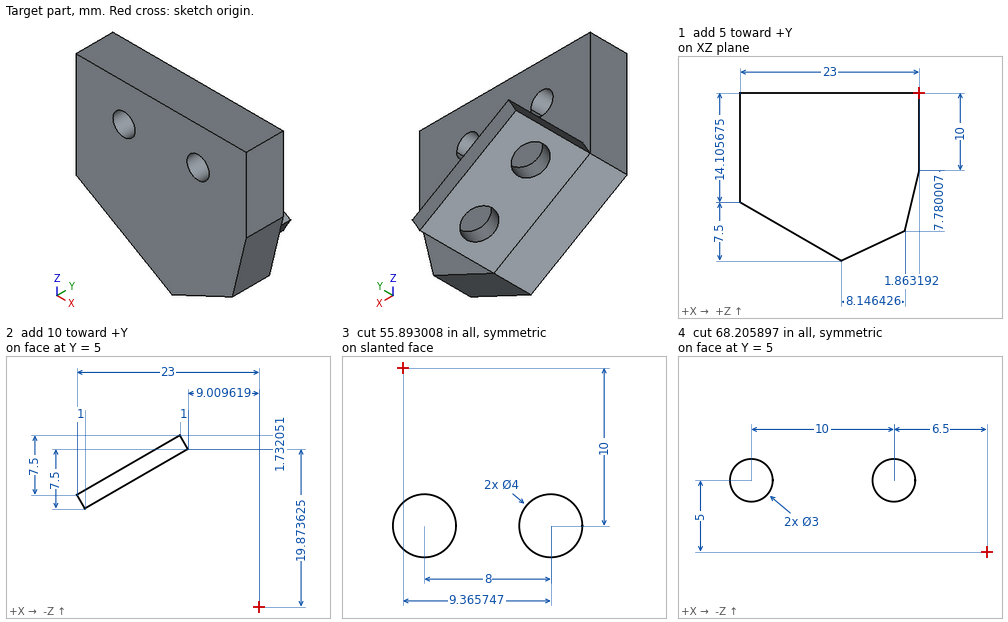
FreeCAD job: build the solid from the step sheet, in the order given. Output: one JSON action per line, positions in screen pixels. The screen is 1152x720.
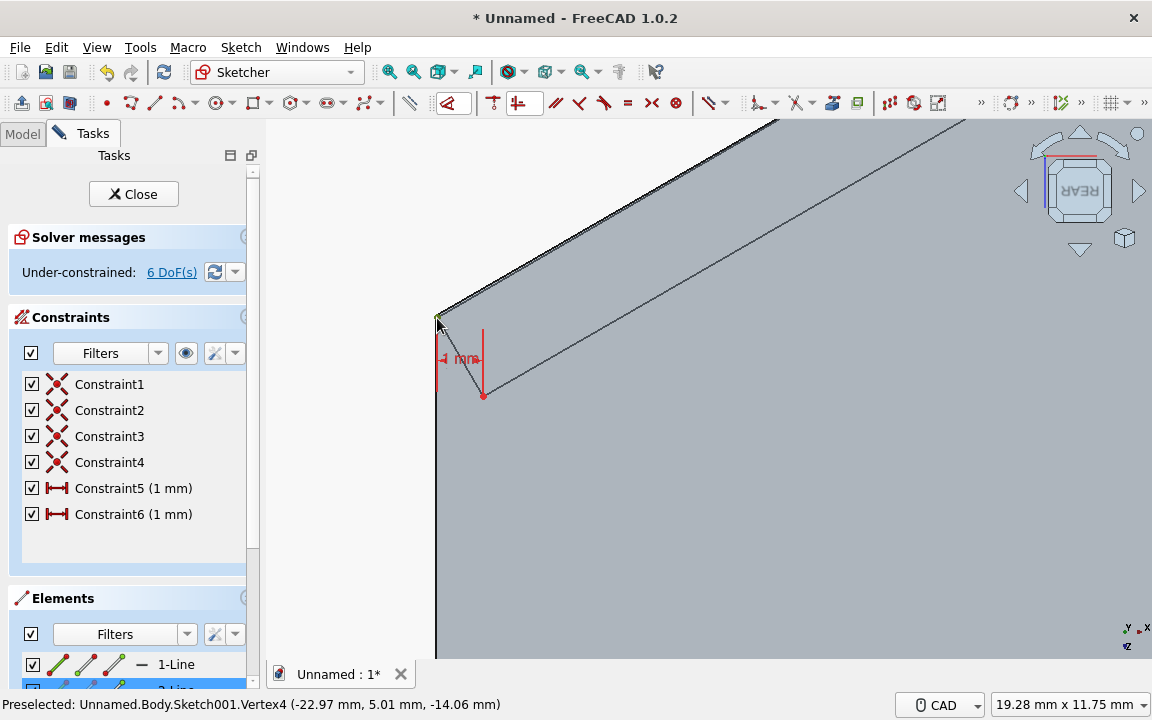
{"action": "key", "text": "l"}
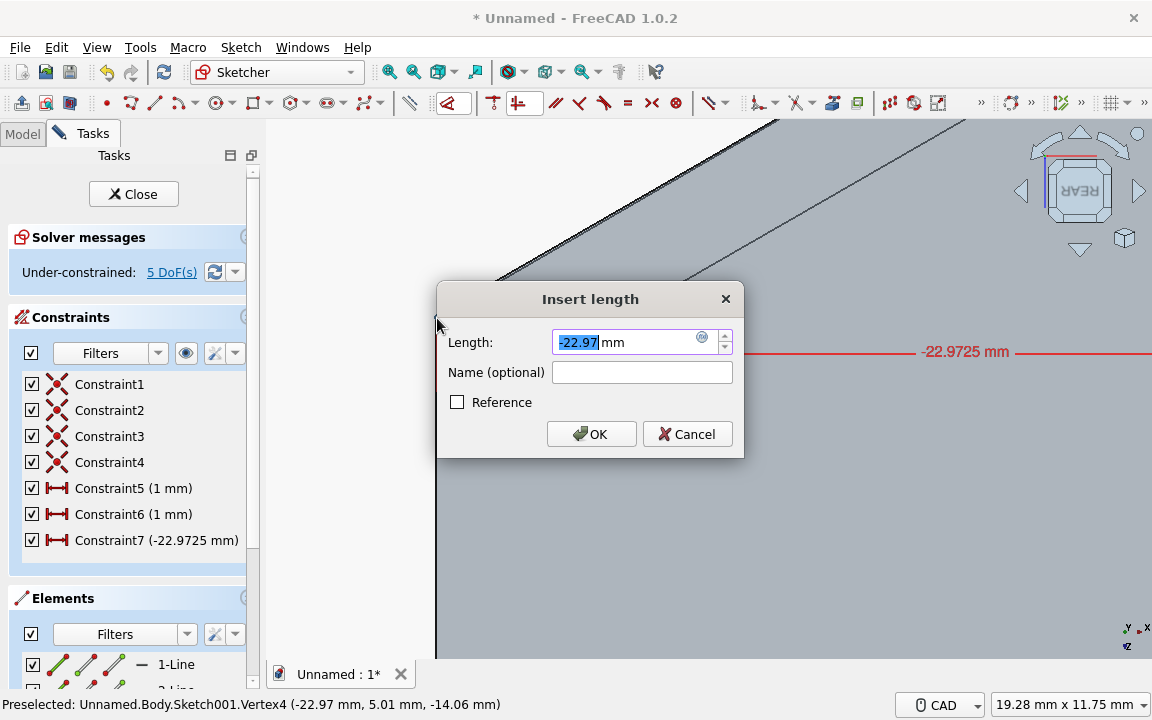
{"action": "type", "text": "-23"}
{"action": "key", "text": "Return"}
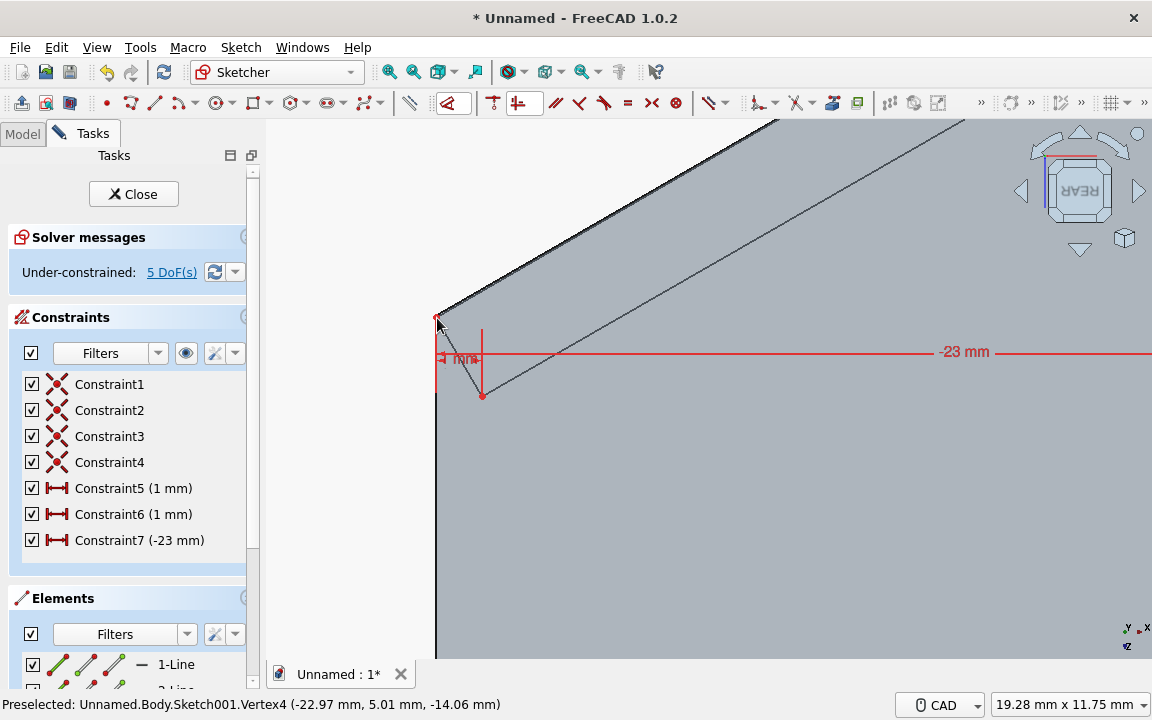
{"action": "left_click", "coordinate": [615, 214]}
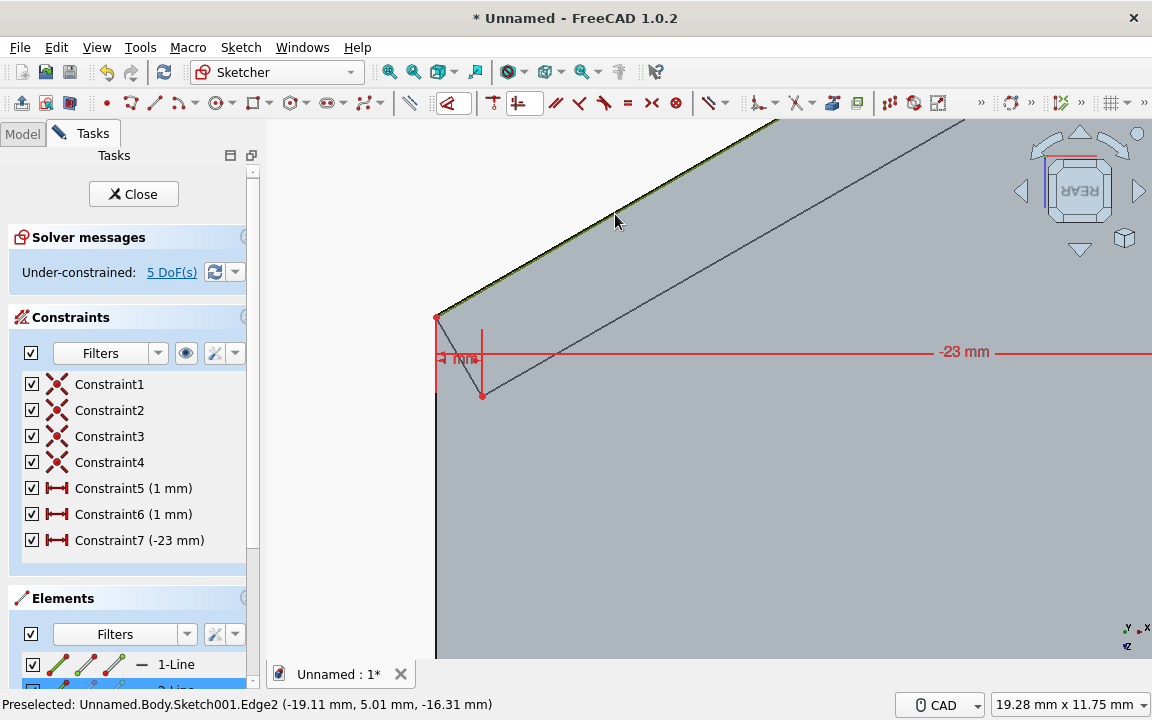
{"action": "left_click", "coordinate": [466, 104]}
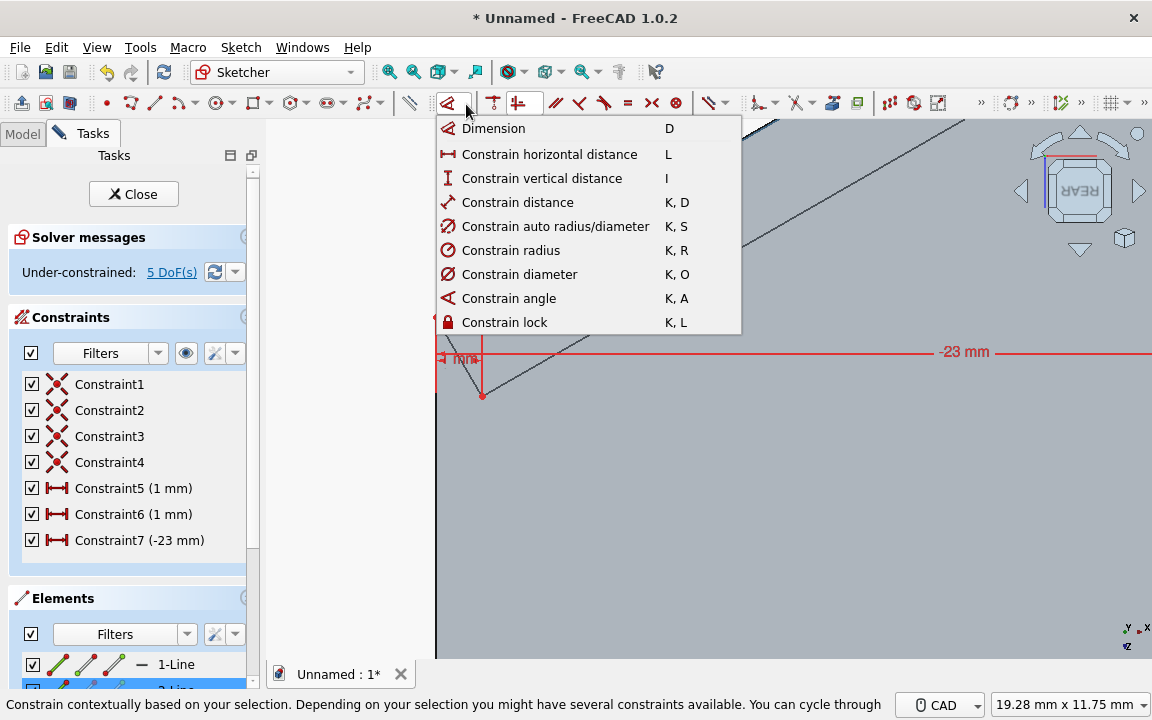
{"action": "left_click", "coordinate": [589, 178]}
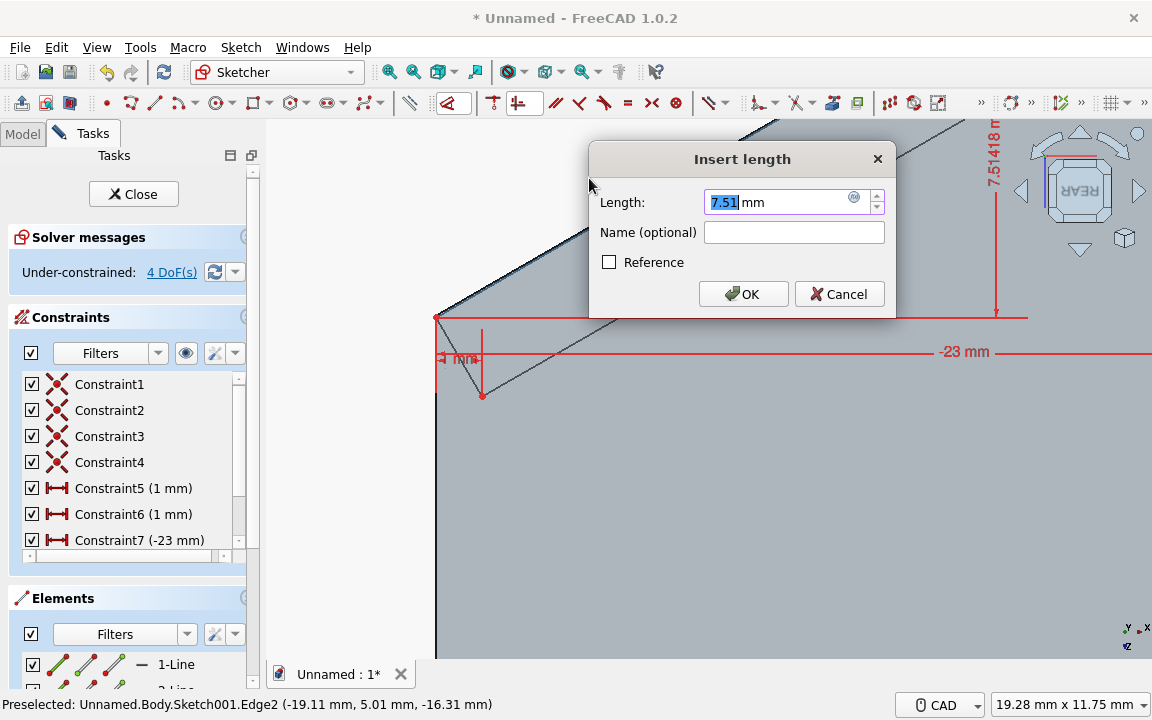
{"action": "type", "text": "7.5"}
{"action": "key", "text": "Return"}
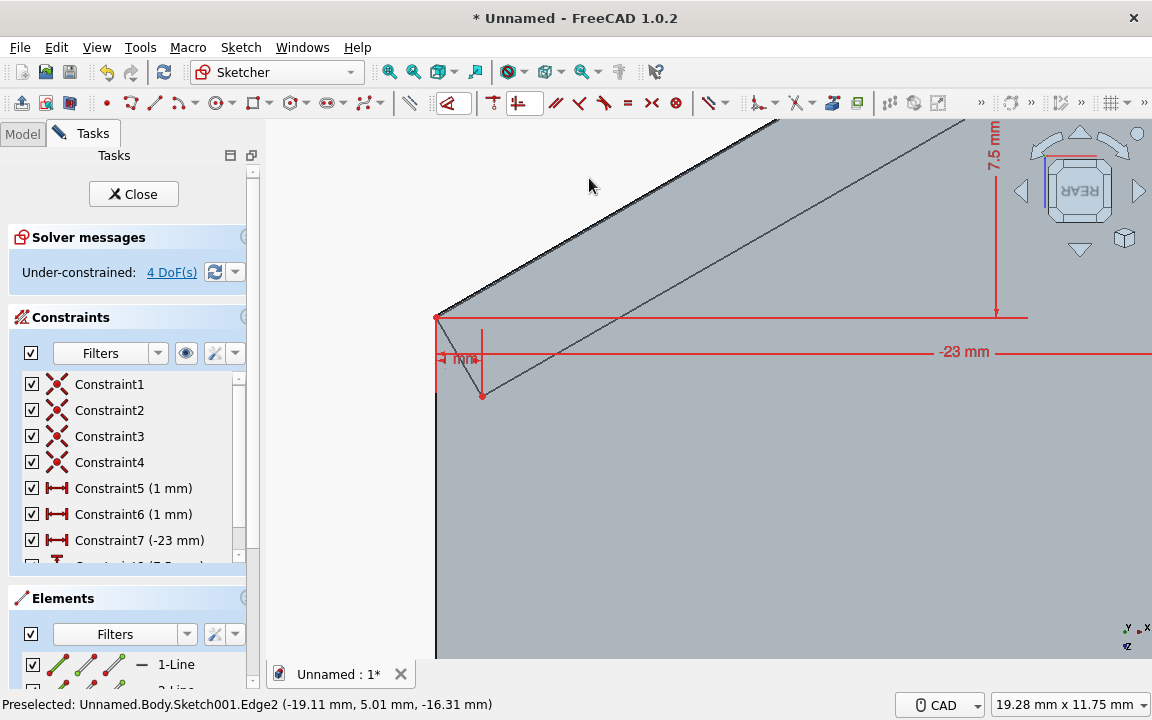
{"action": "left_click", "coordinate": [661, 294]}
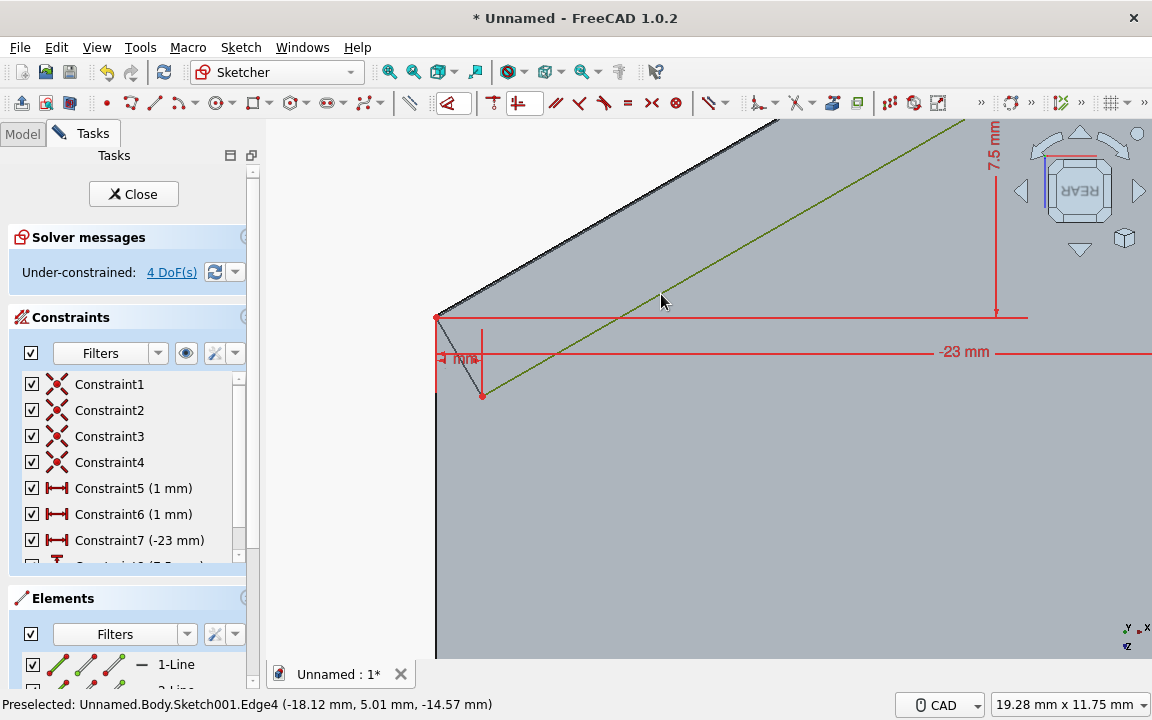
{"action": "key", "text": "i"}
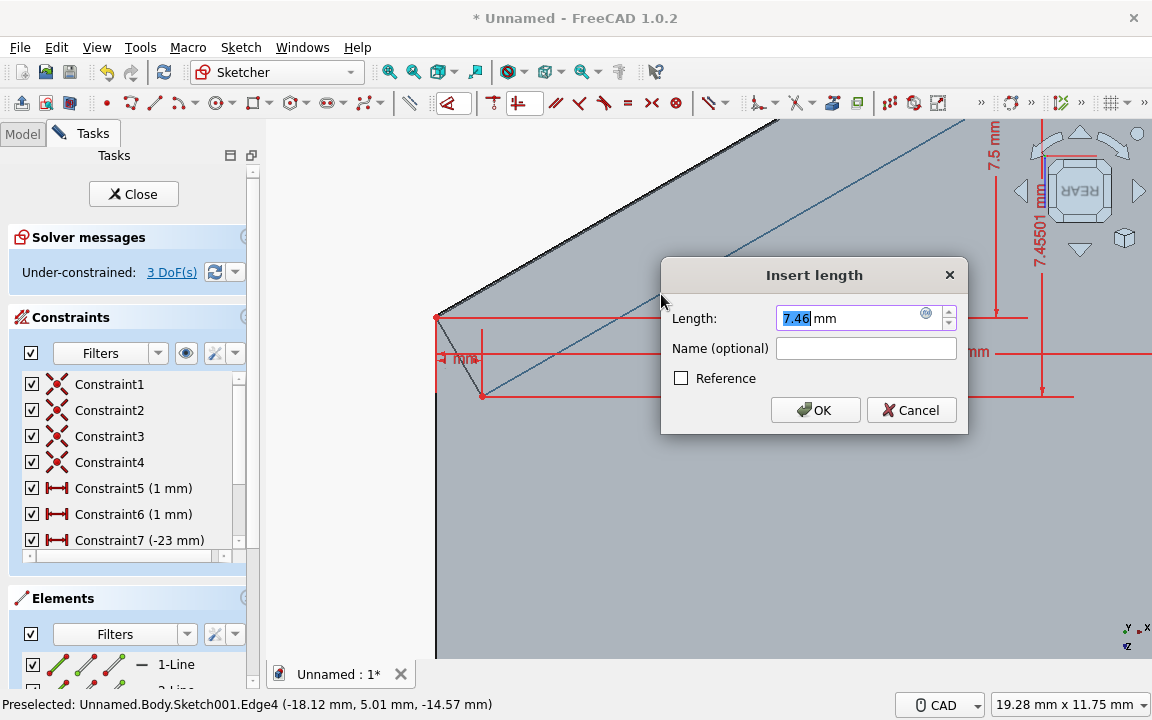
{"action": "type", "text": "7.5"}
{"action": "key", "text": "Return"}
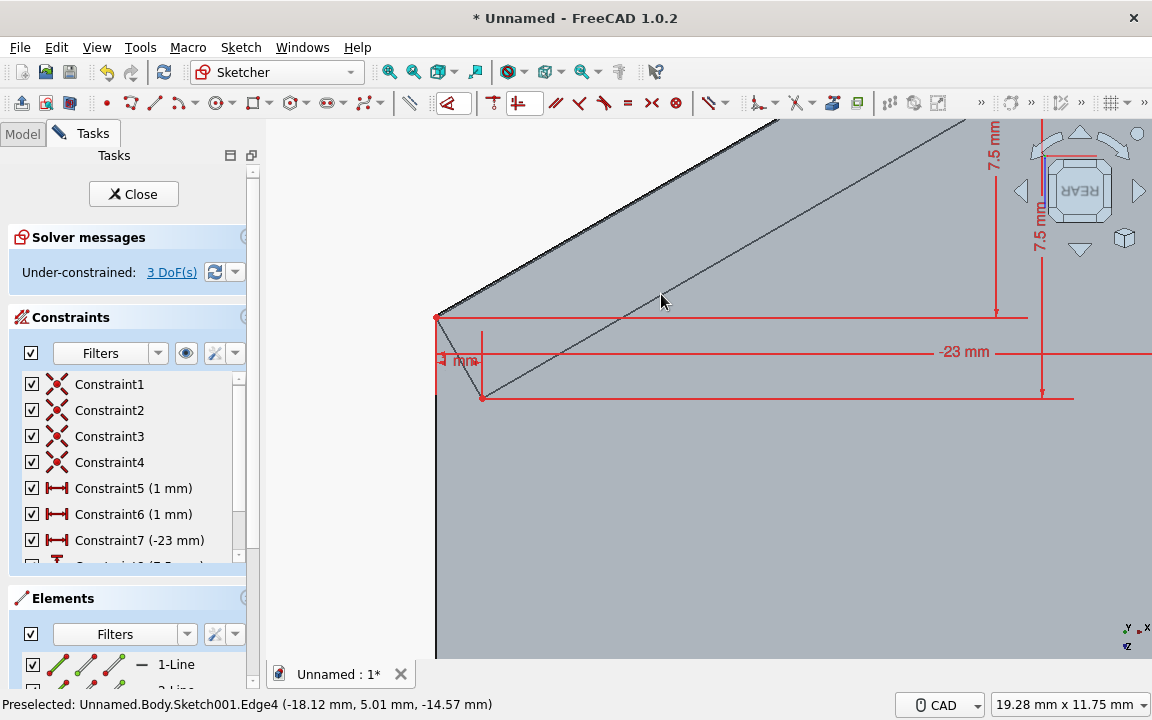
{"action": "scroll", "coordinate": [452, 343], "scroll_direction": "down", "scroll_amount": 5}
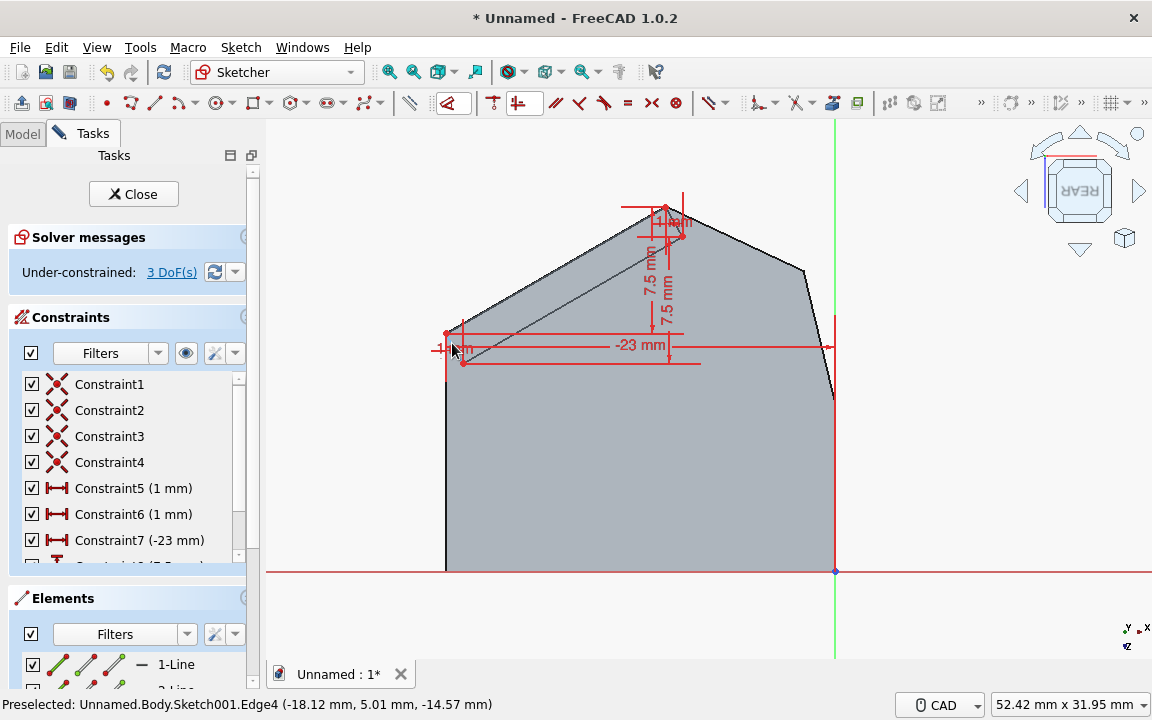
{"action": "left_click", "coordinate": [683, 237]}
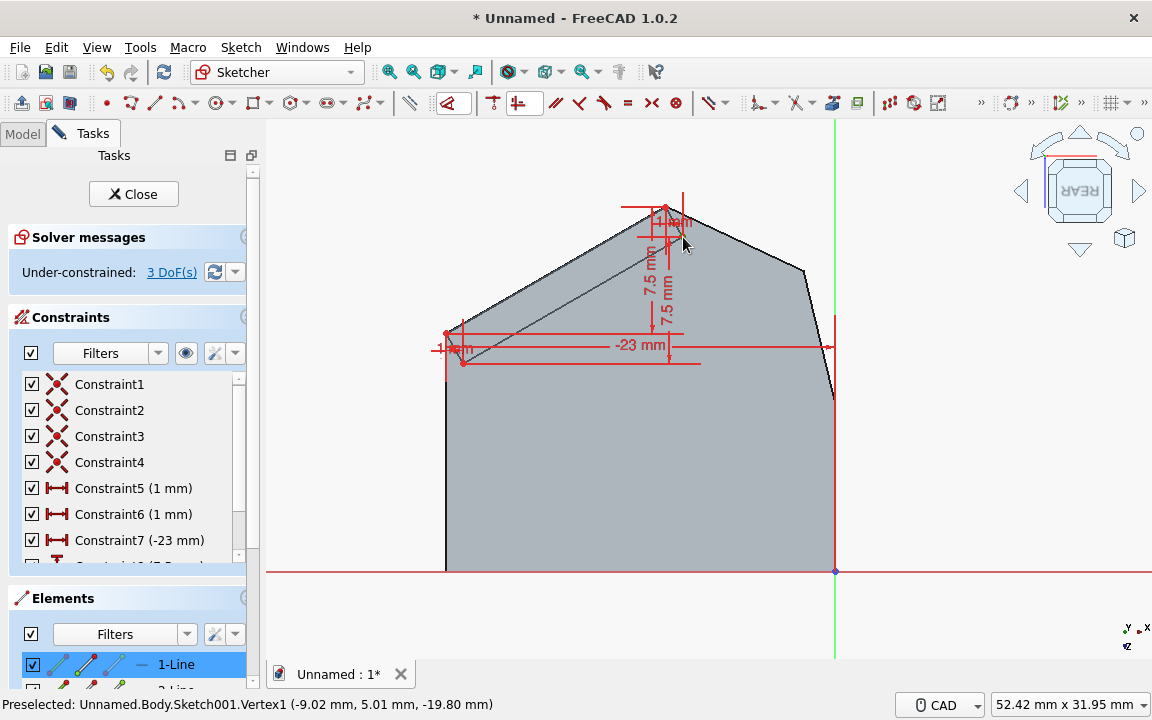
{"action": "key", "text": "l"}